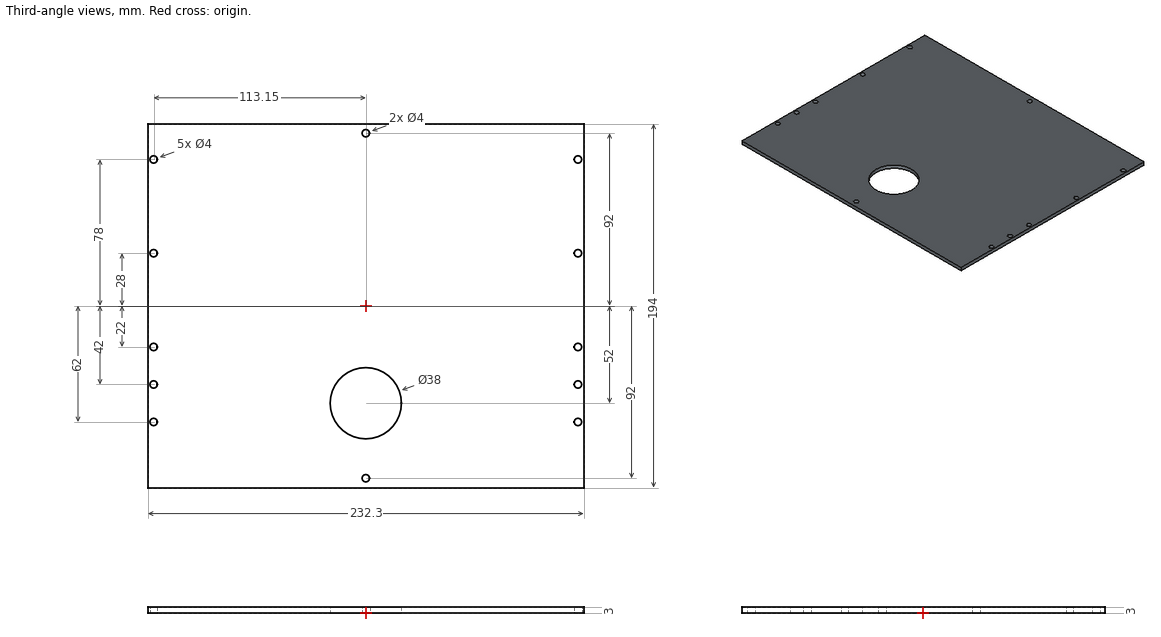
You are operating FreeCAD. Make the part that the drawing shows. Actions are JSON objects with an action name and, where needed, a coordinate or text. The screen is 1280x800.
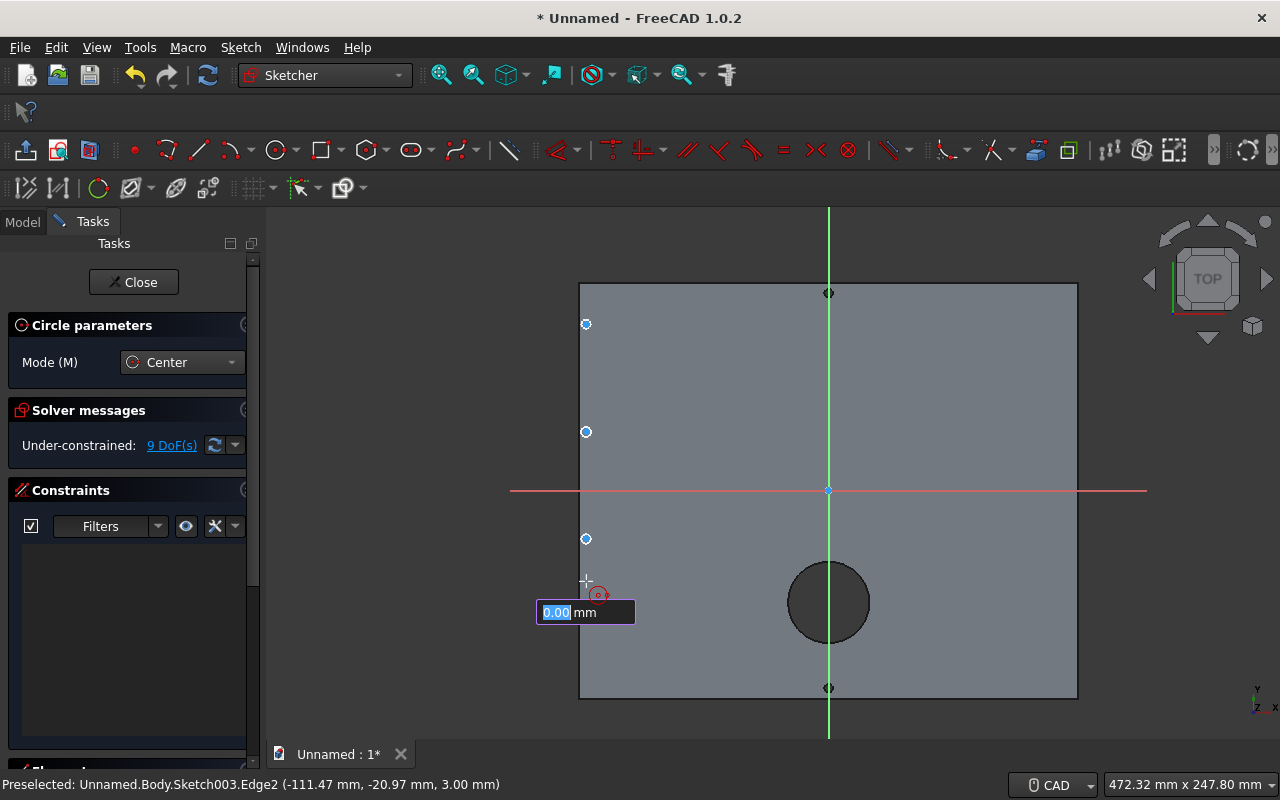
{"action": "scroll", "coordinate": [589, 578], "scroll_direction": "up", "scroll_amount": 7}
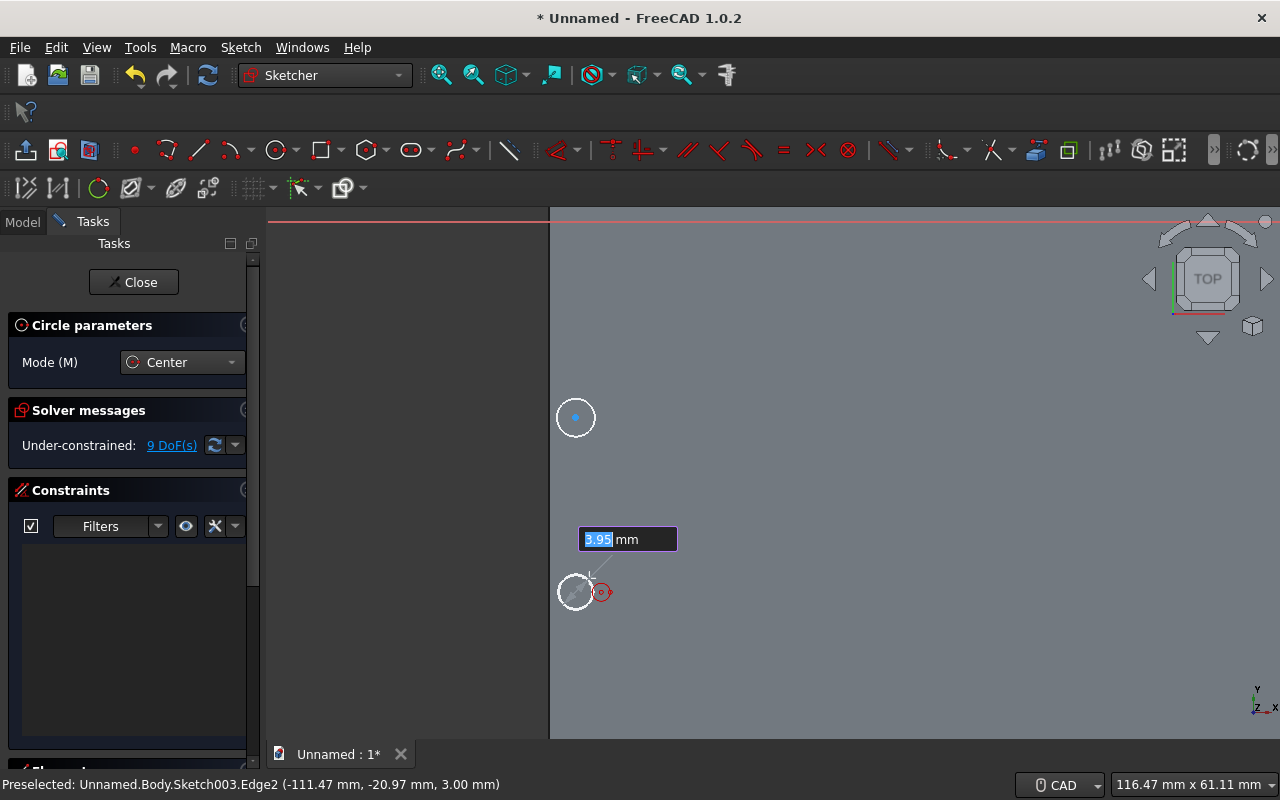
{"action": "left_click", "coordinate": [587, 576]}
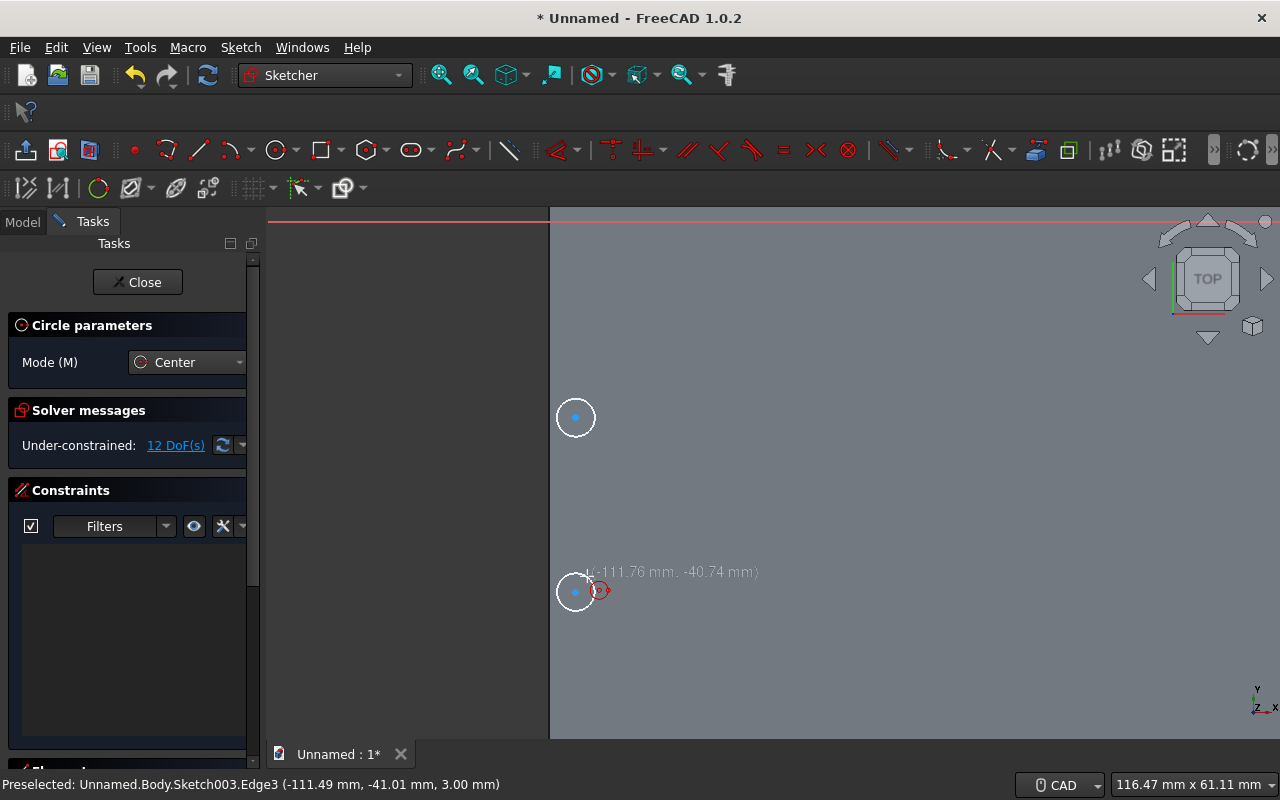
{"action": "scroll", "coordinate": [589, 578], "scroll_direction": "down", "scroll_amount": 7}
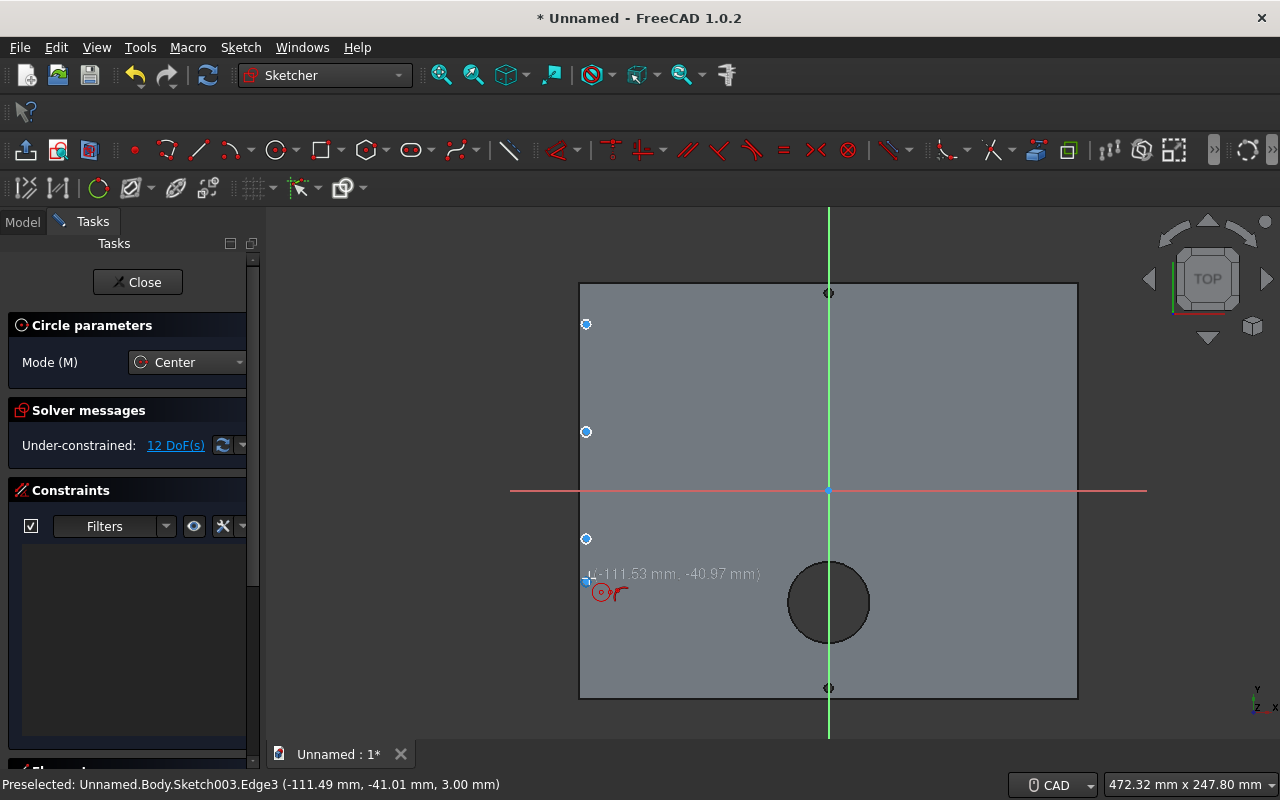
{"action": "scroll", "coordinate": [586, 624], "scroll_direction": "up", "scroll_amount": 9}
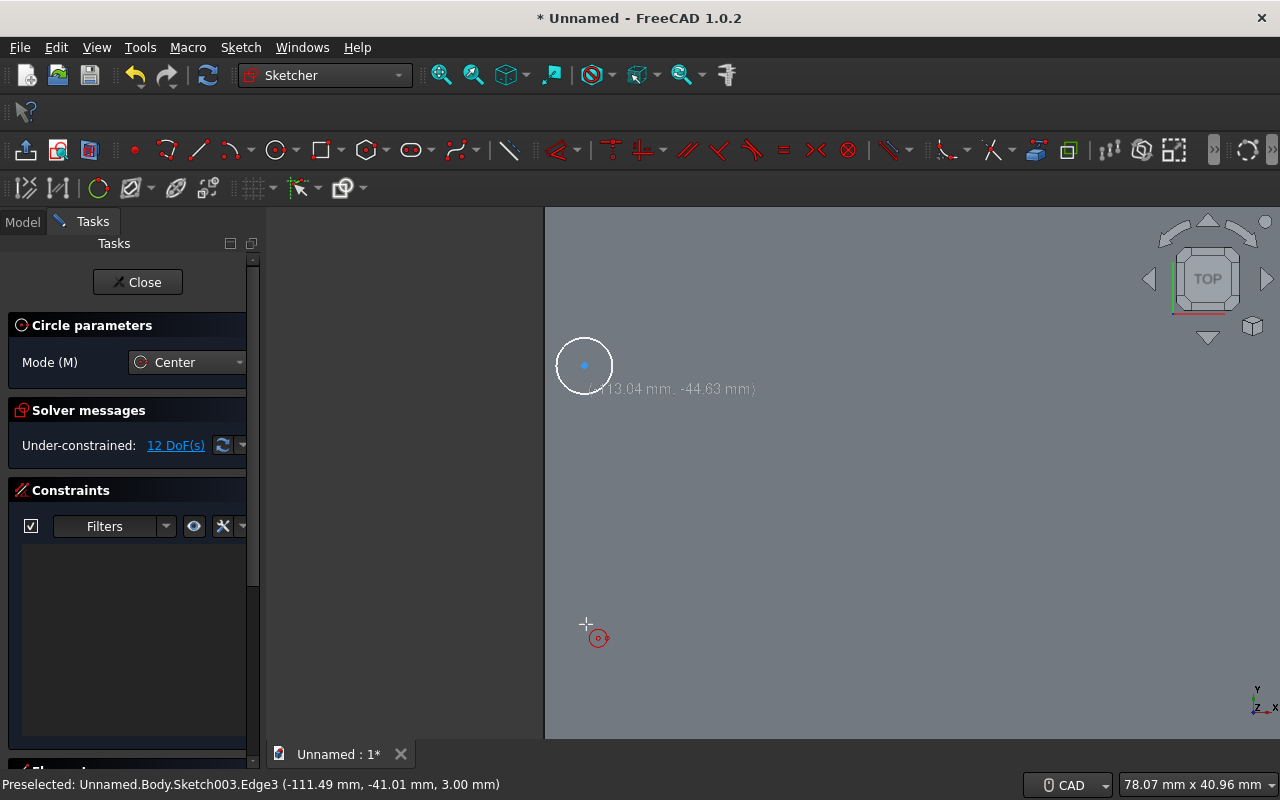
{"action": "scroll", "coordinate": [586, 624], "scroll_direction": "down", "scroll_amount": 9}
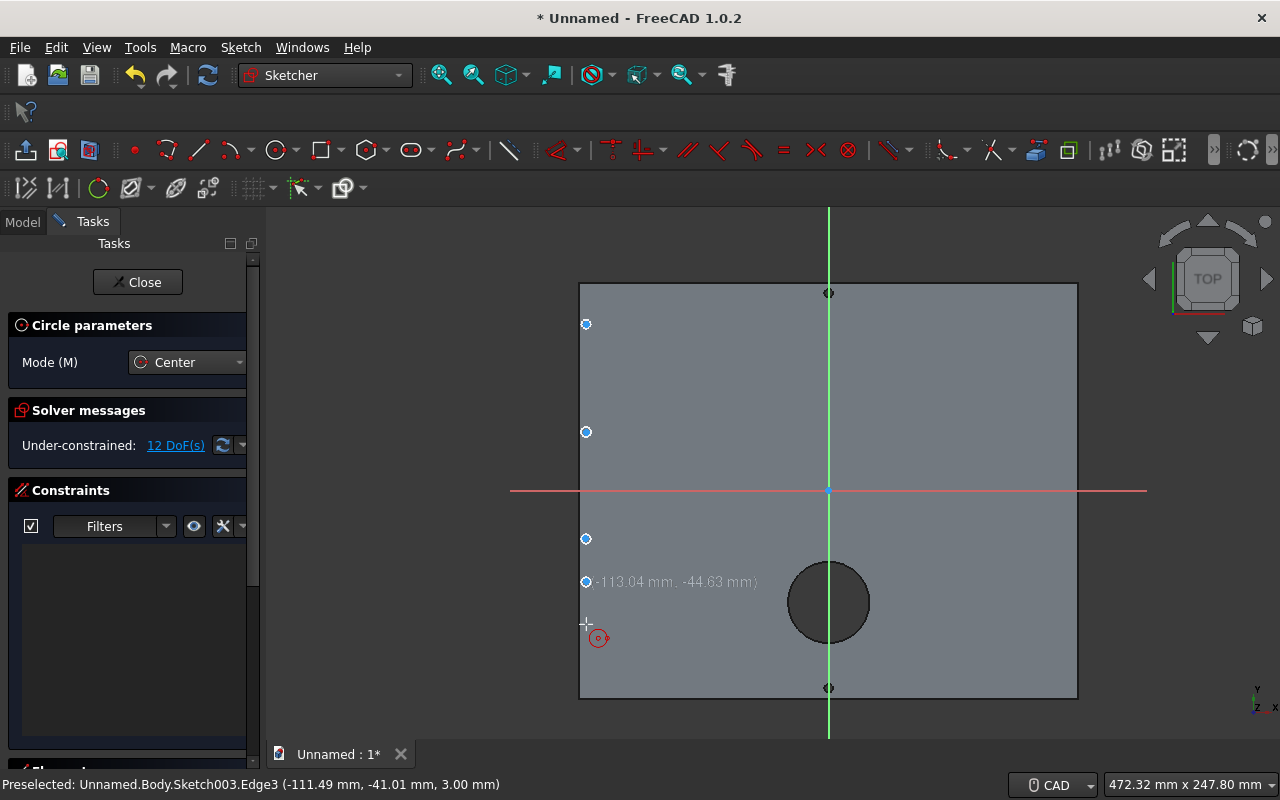
{"action": "left_click", "coordinate": [586, 624]}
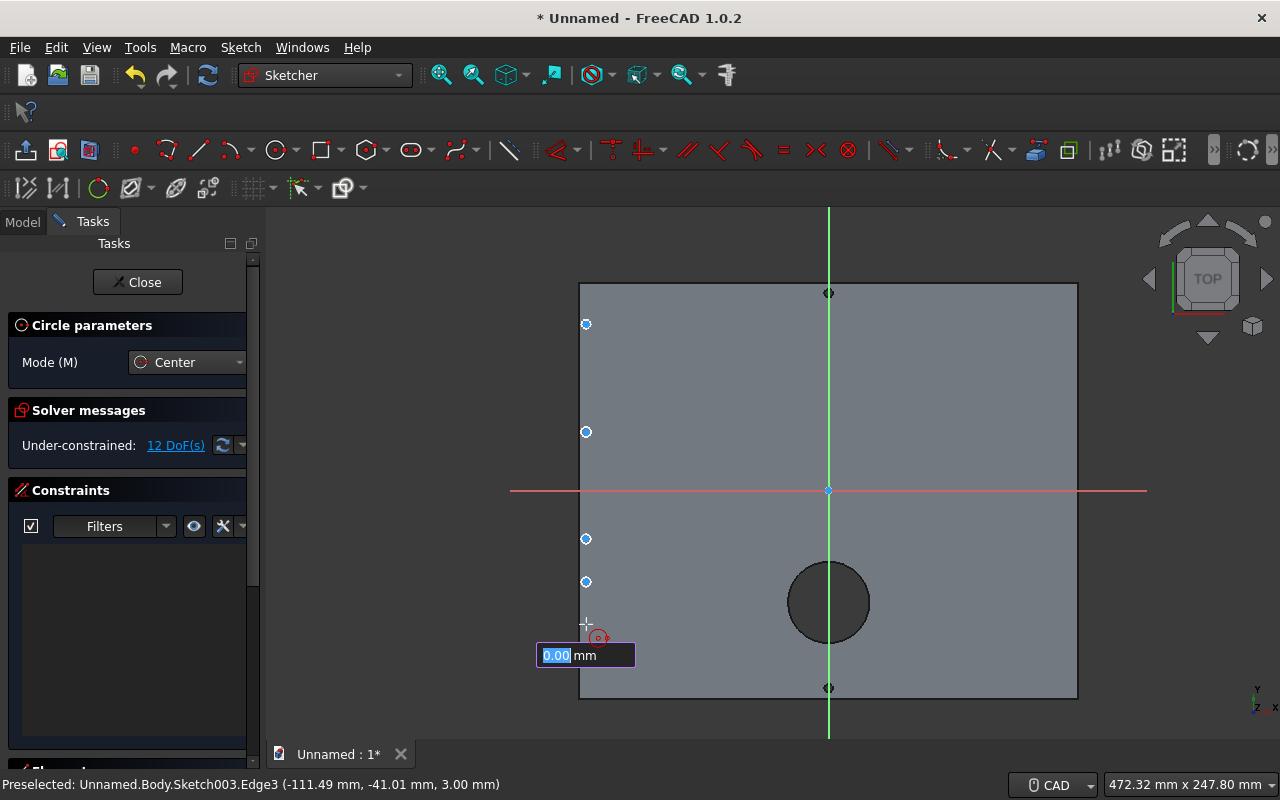
{"action": "scroll", "coordinate": [589, 621], "scroll_direction": "up", "scroll_amount": 7}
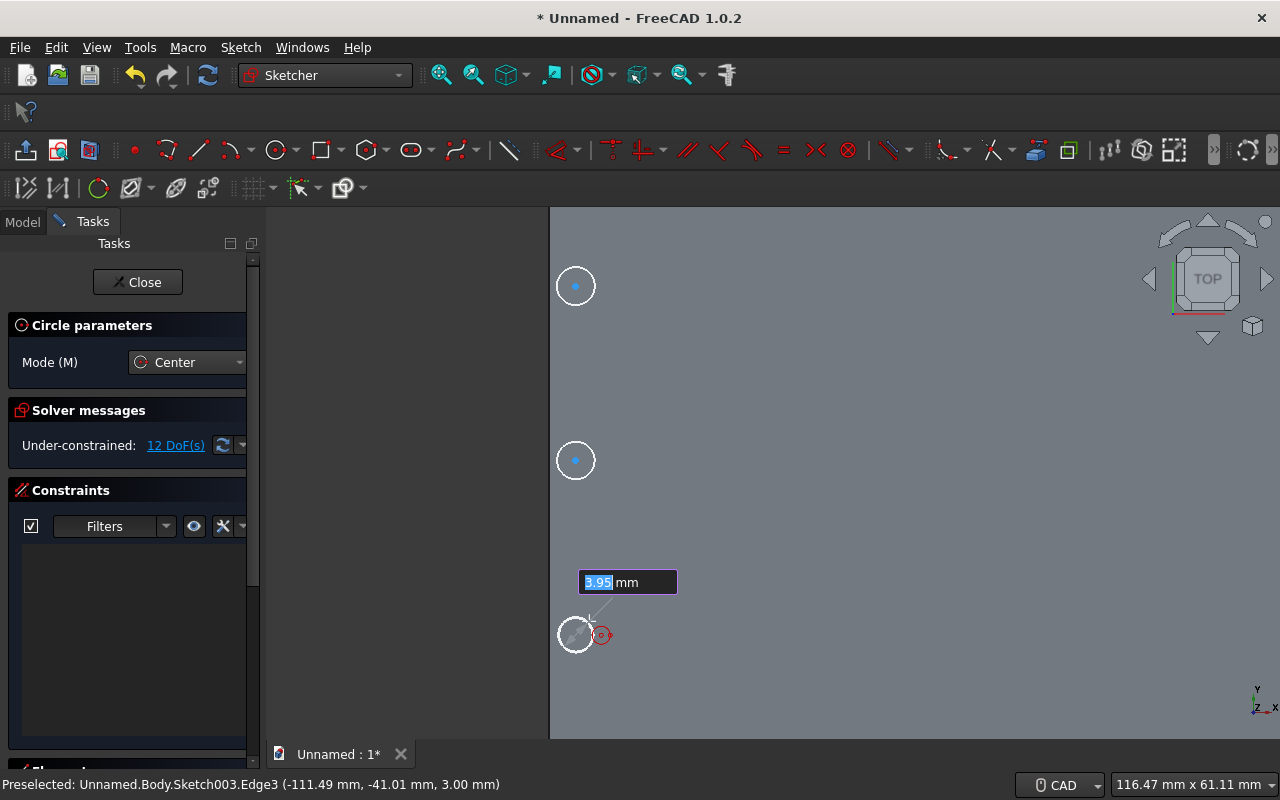
{"action": "left_click", "coordinate": [587, 618]}
{"action": "key", "text": "Escape"}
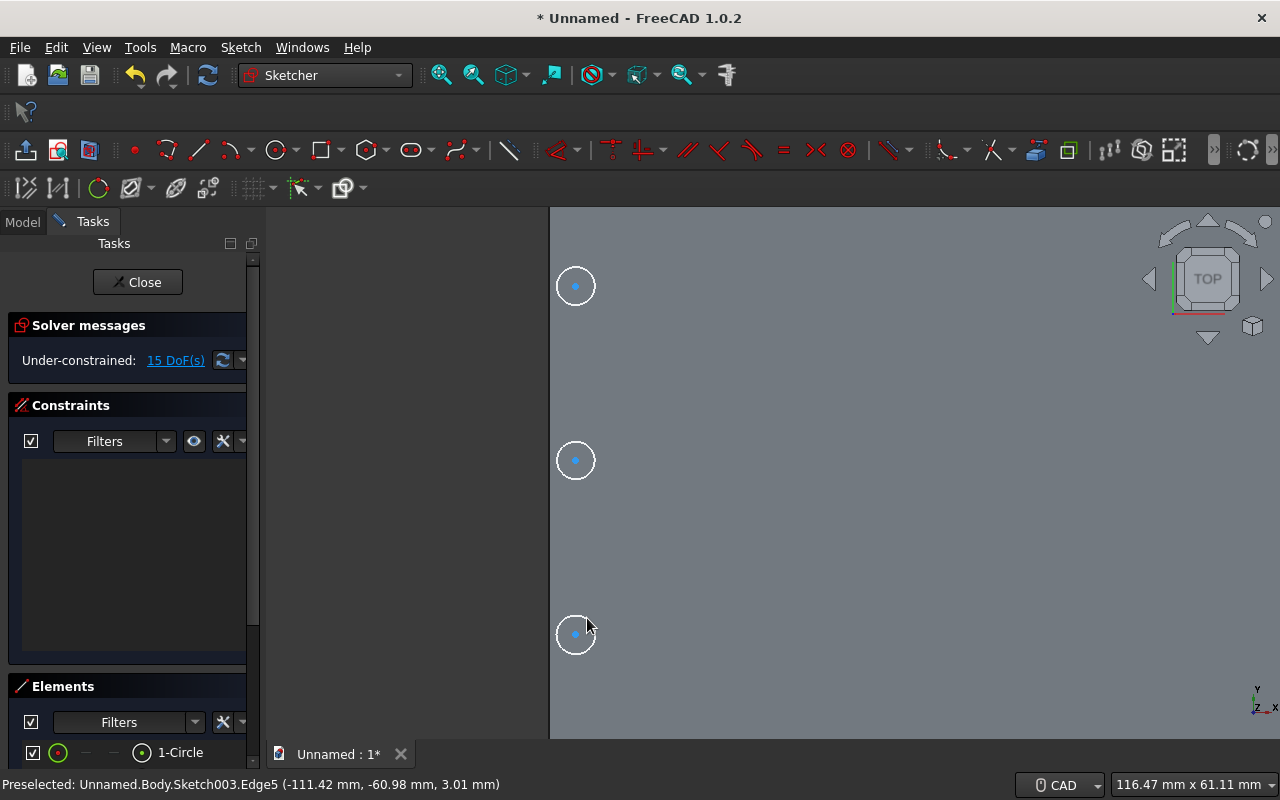
{"action": "scroll", "coordinate": [589, 621], "scroll_direction": "down", "scroll_amount": 7}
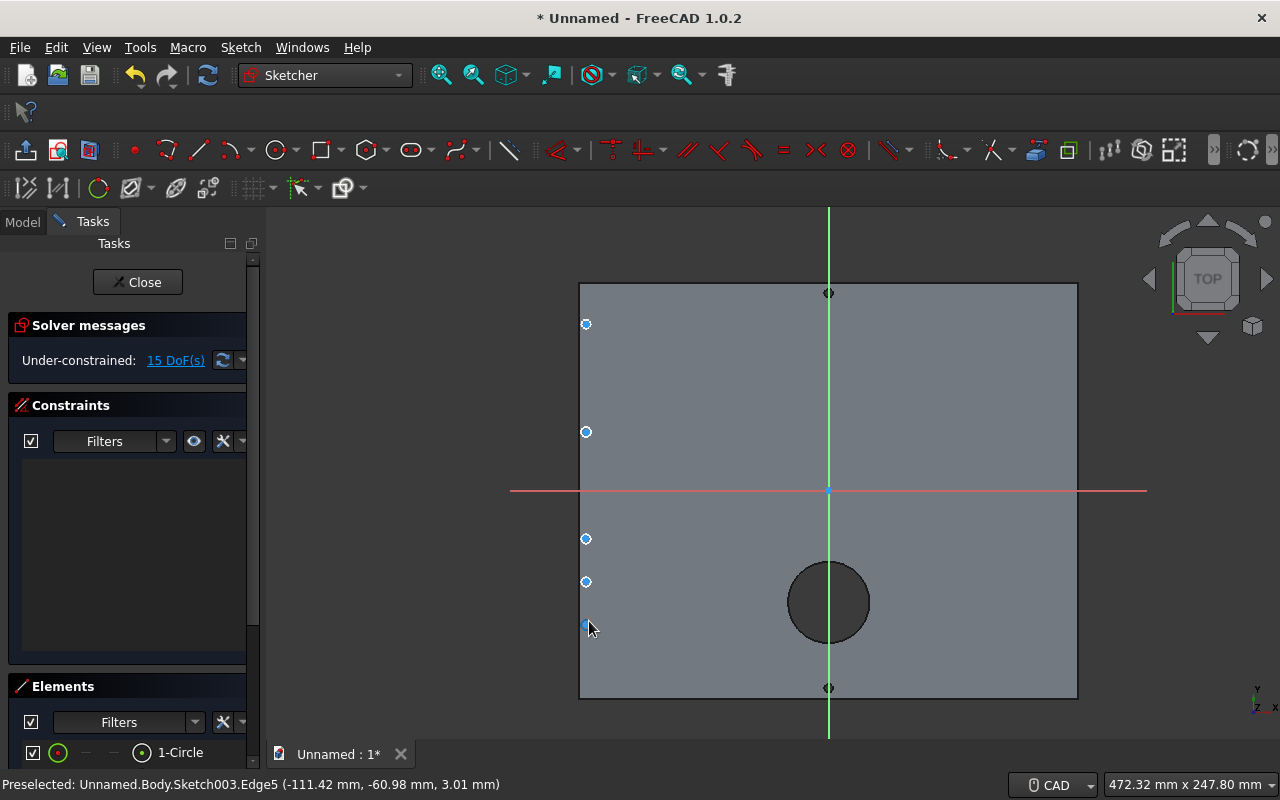
{"action": "scroll", "coordinate": [589, 321], "scroll_direction": "up", "scroll_amount": 6}